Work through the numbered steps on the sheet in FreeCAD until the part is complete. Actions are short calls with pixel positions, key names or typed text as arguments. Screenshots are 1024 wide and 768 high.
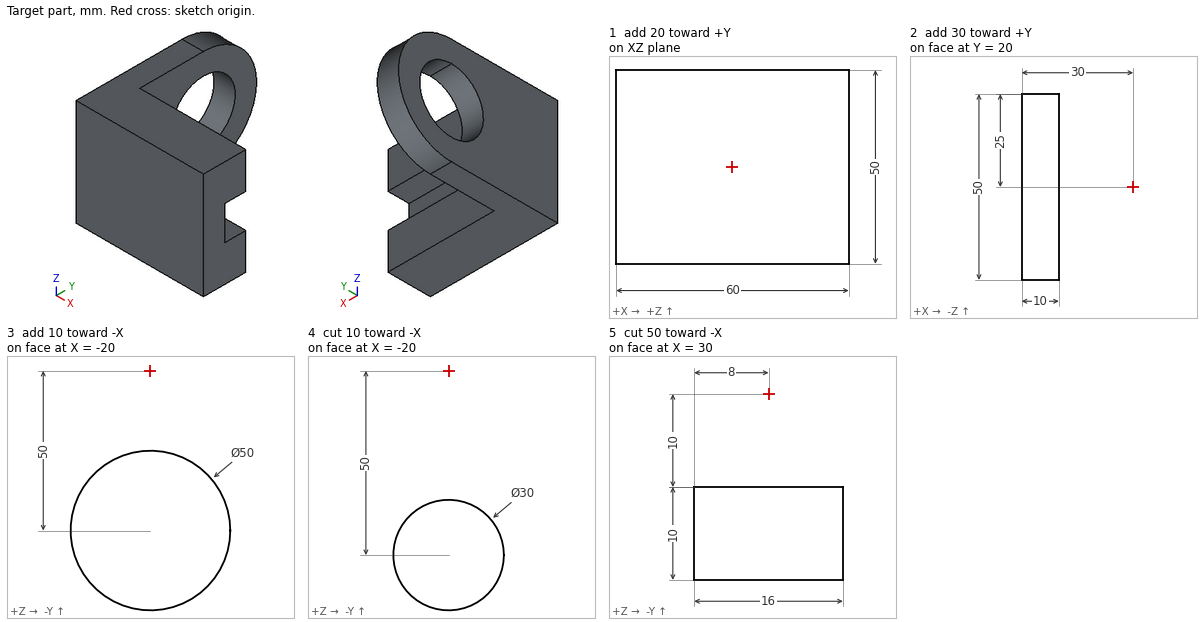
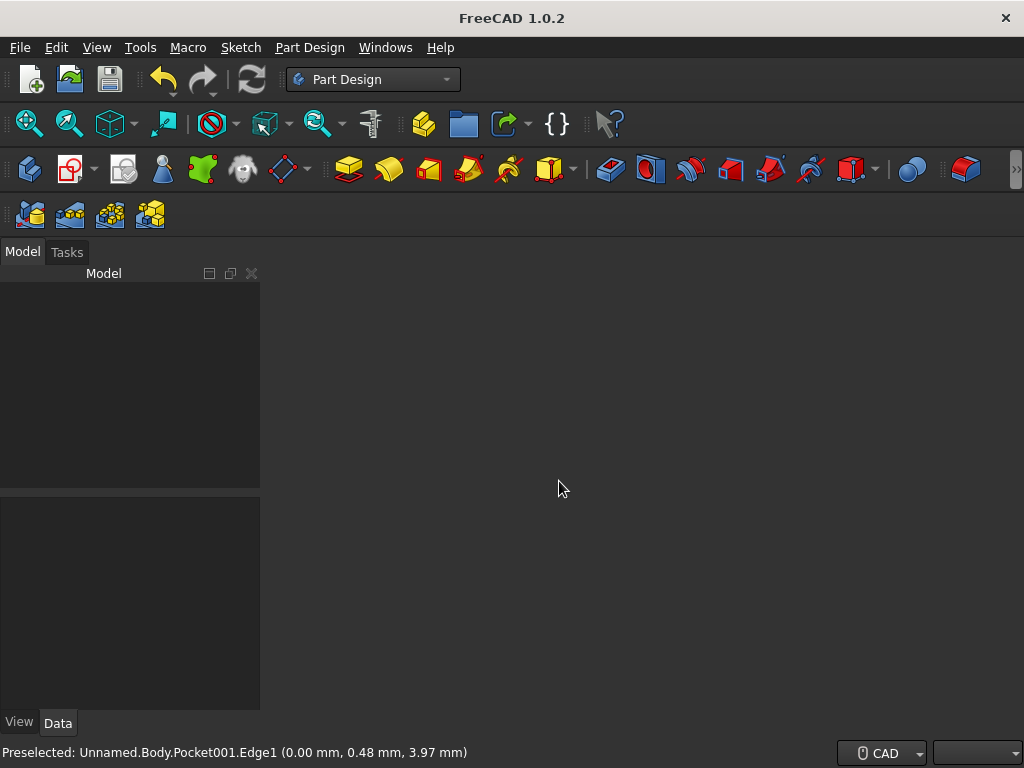
key(ctrl+n)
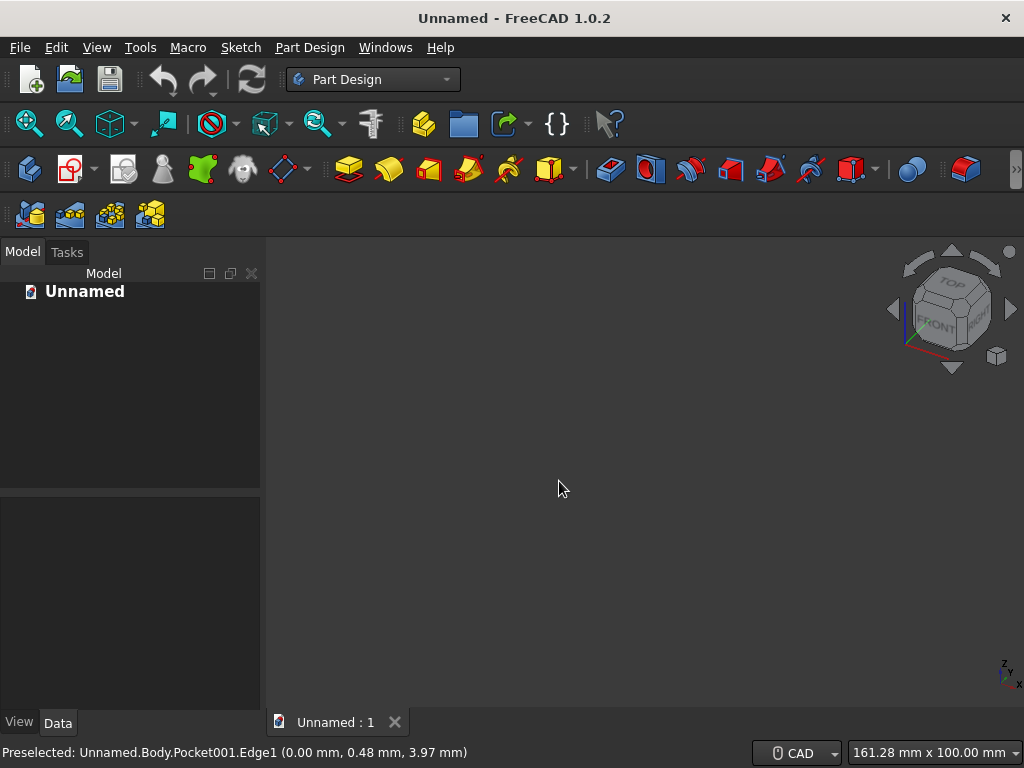
click(70, 170)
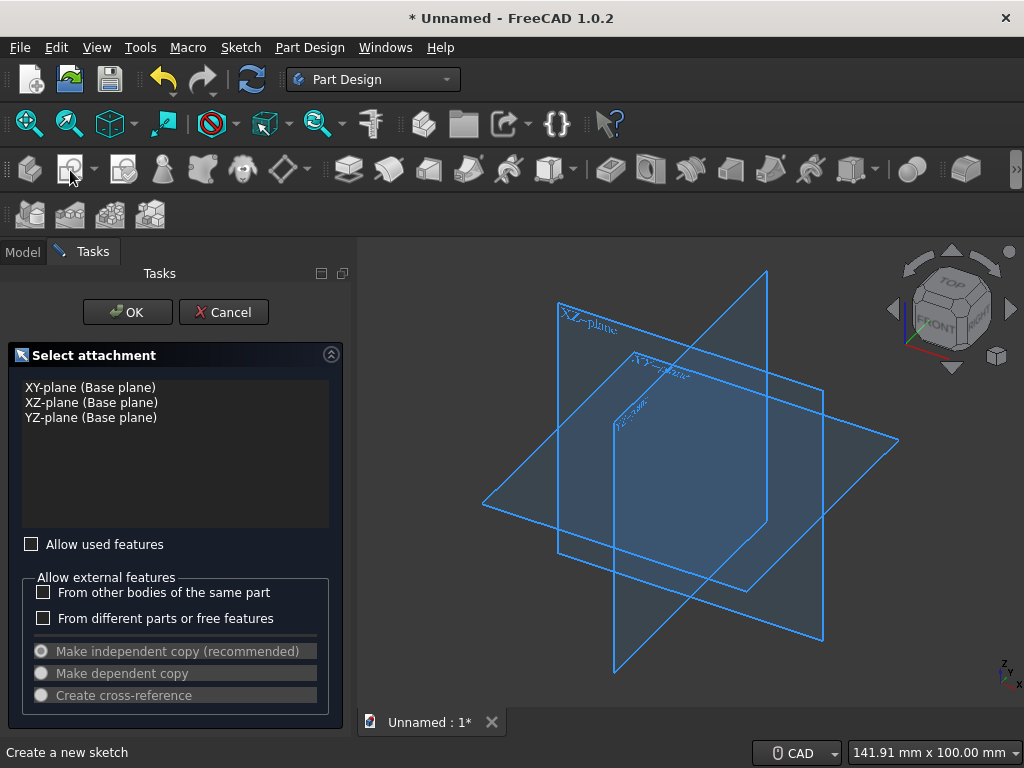
click(82, 402)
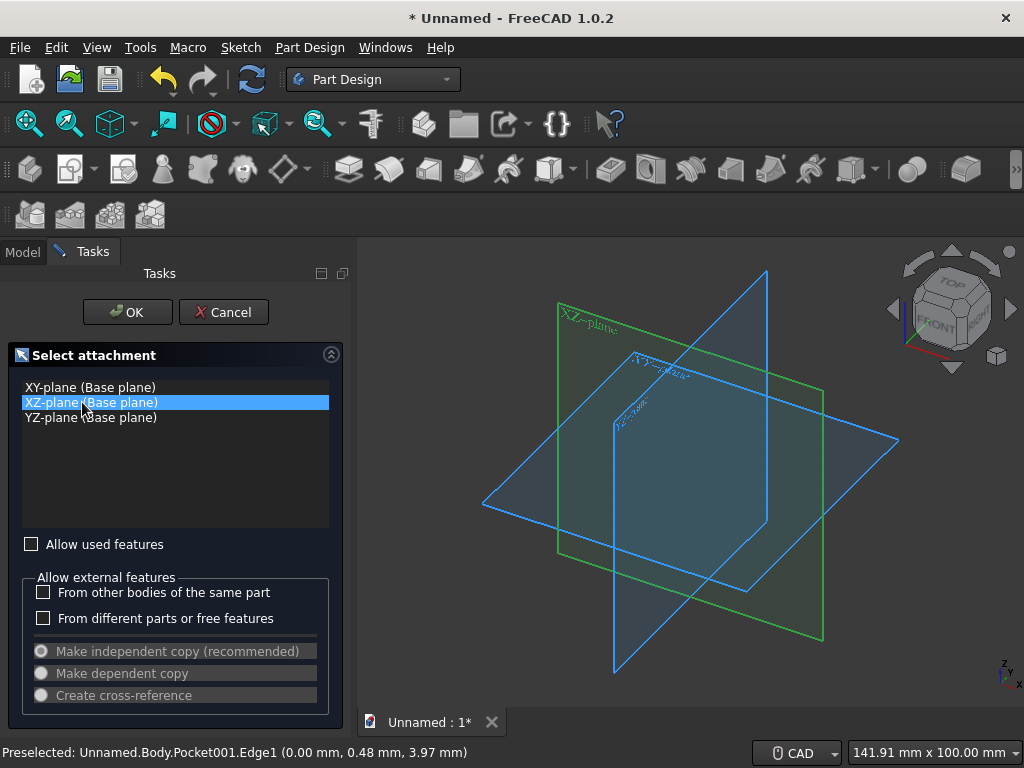
click(128, 312)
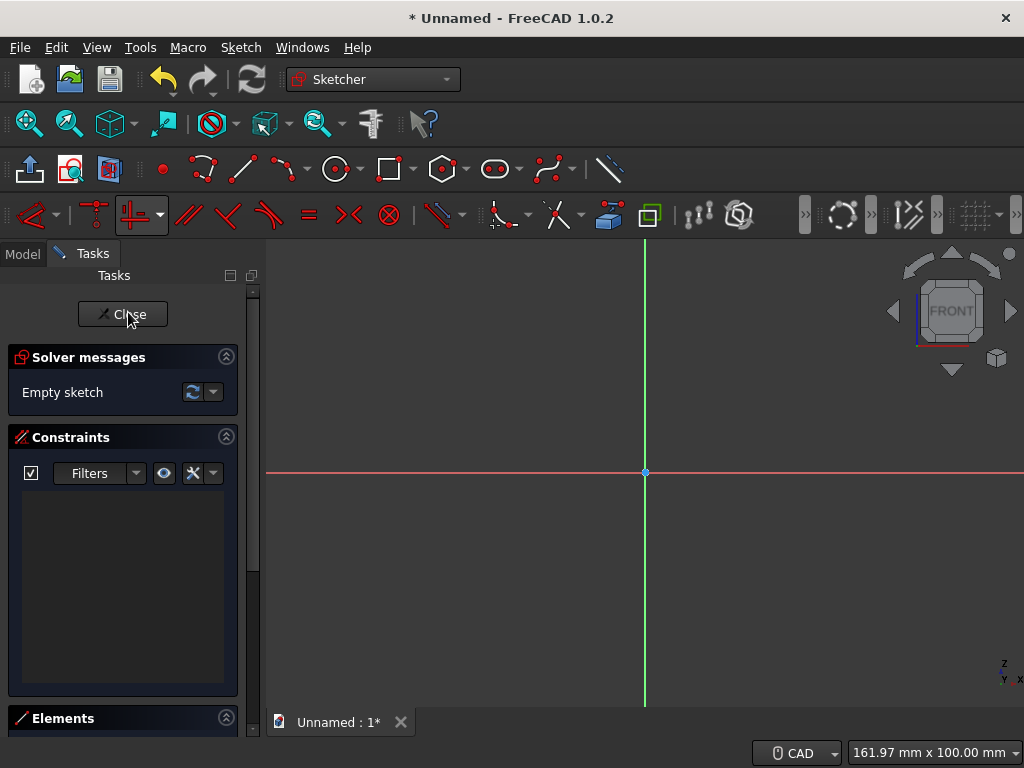
key(g)
key(v)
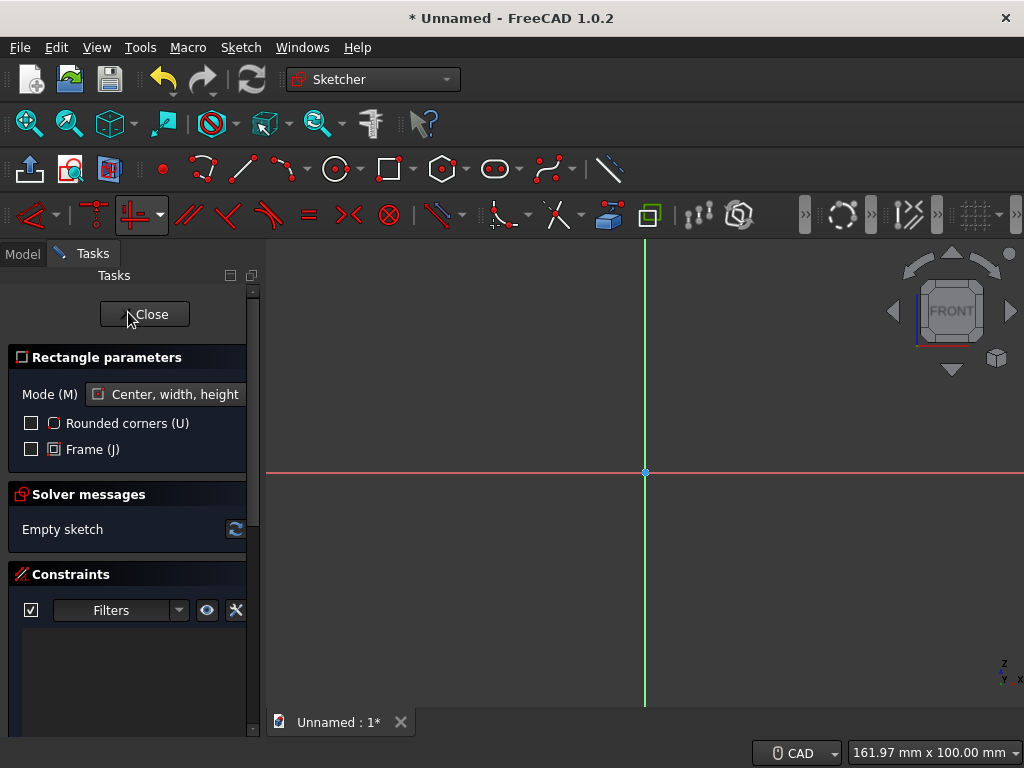
click(645, 473)
click(785, 356)
key(Escape)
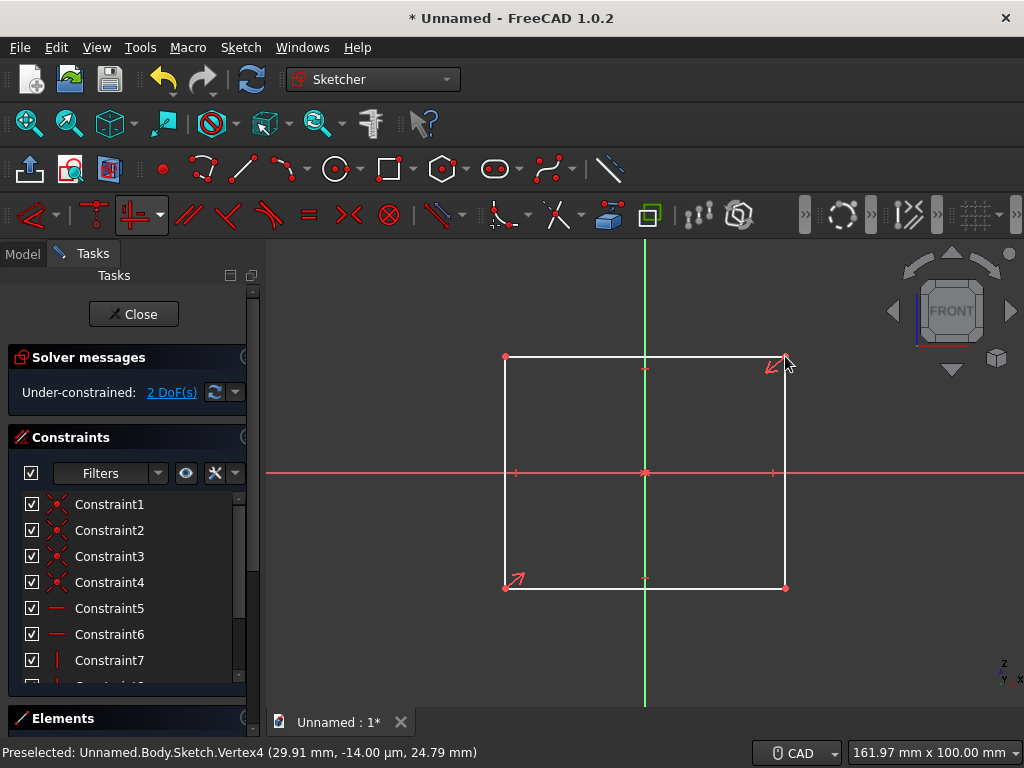
click(32, 216)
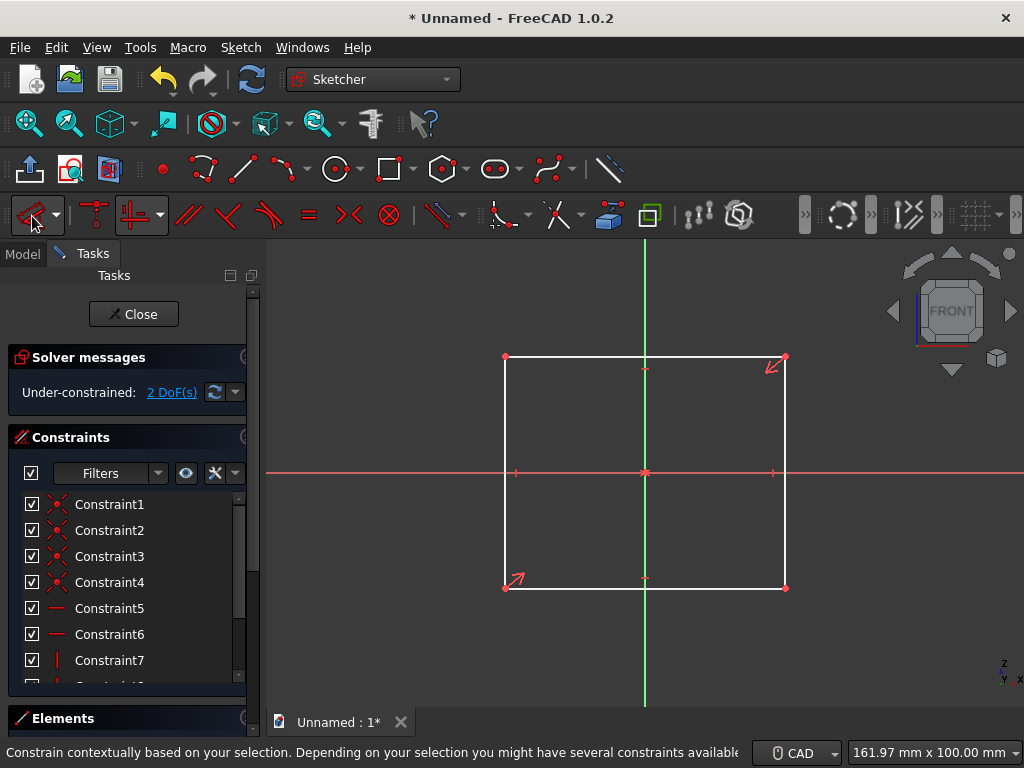
click(589, 589)
click(581, 623)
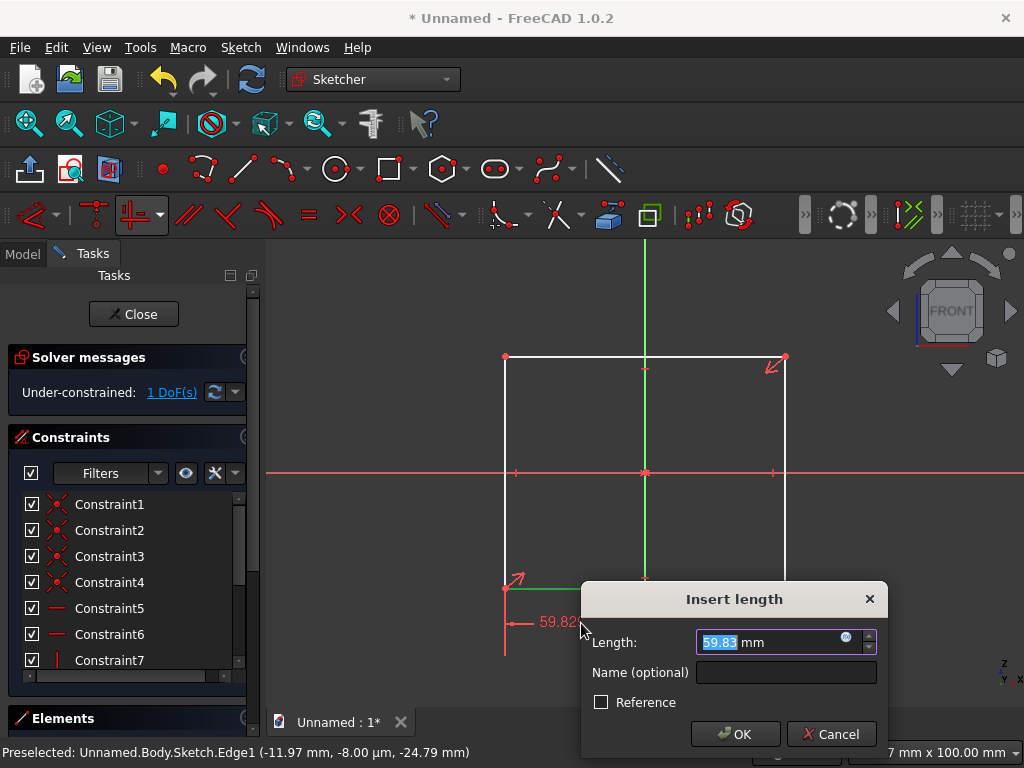
text(60)
key(Return)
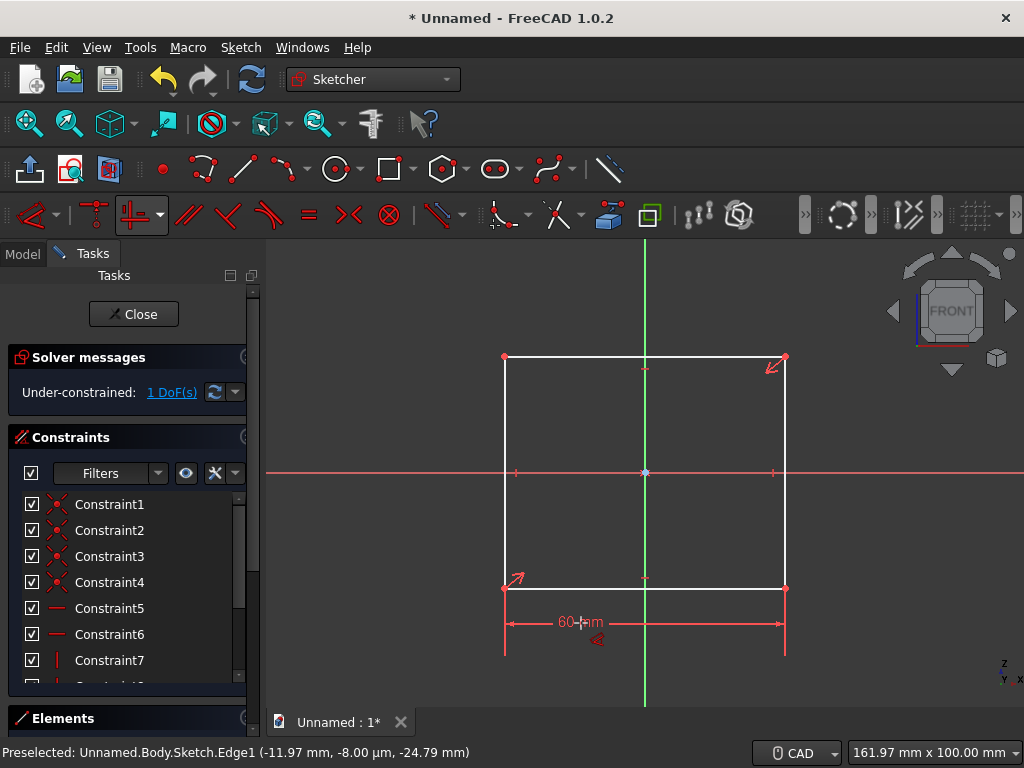
click(785, 519)
click(819, 420)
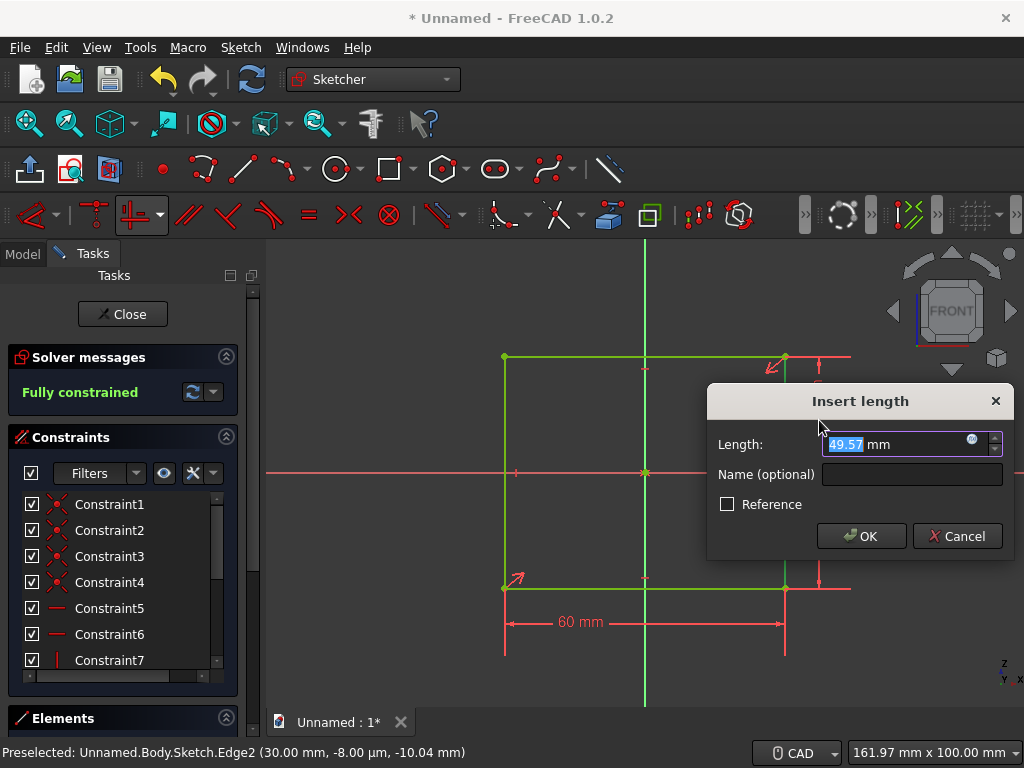
text(50)
key(Return)
key(Escape)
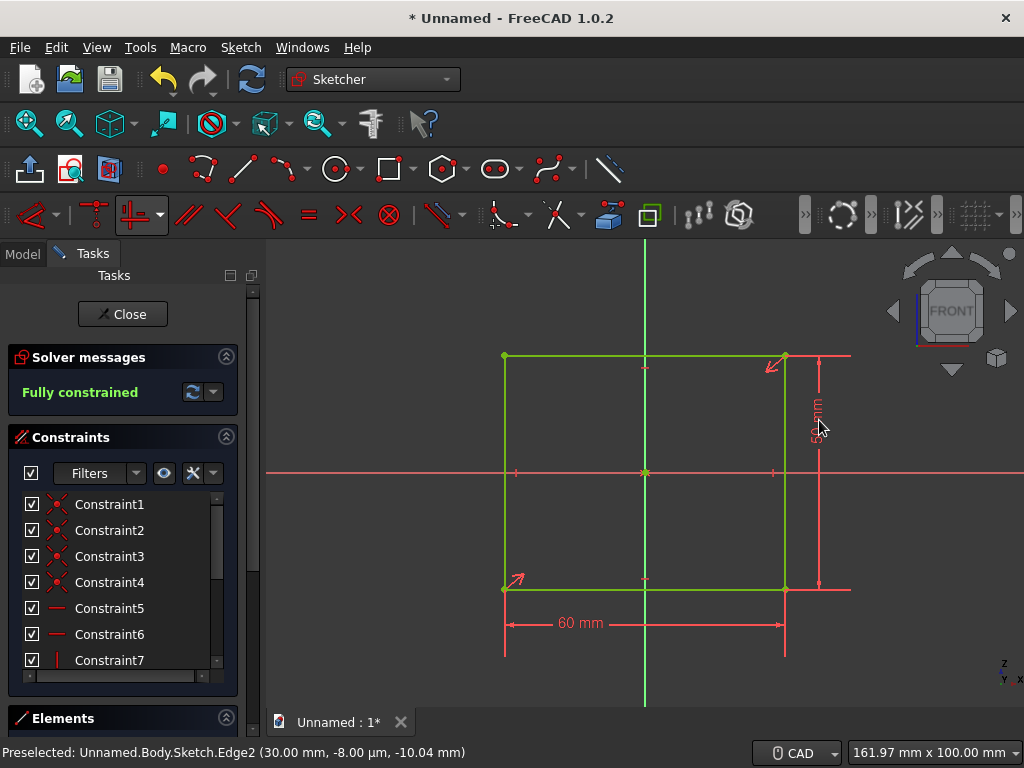
click(123, 314)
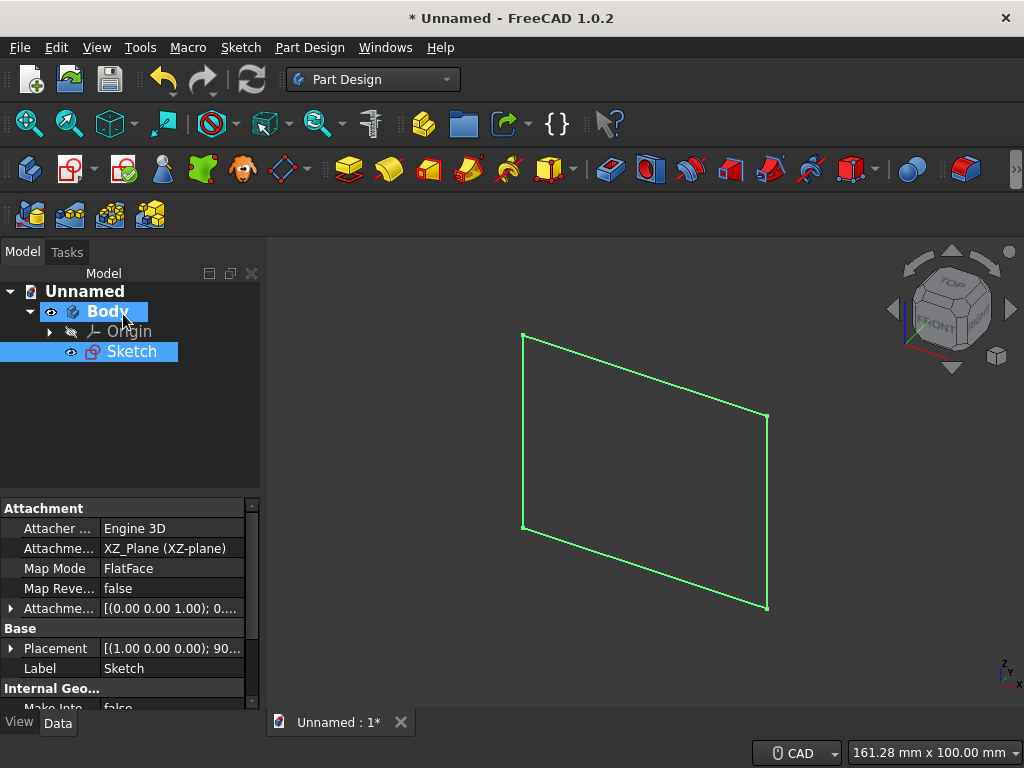
click(350, 170)